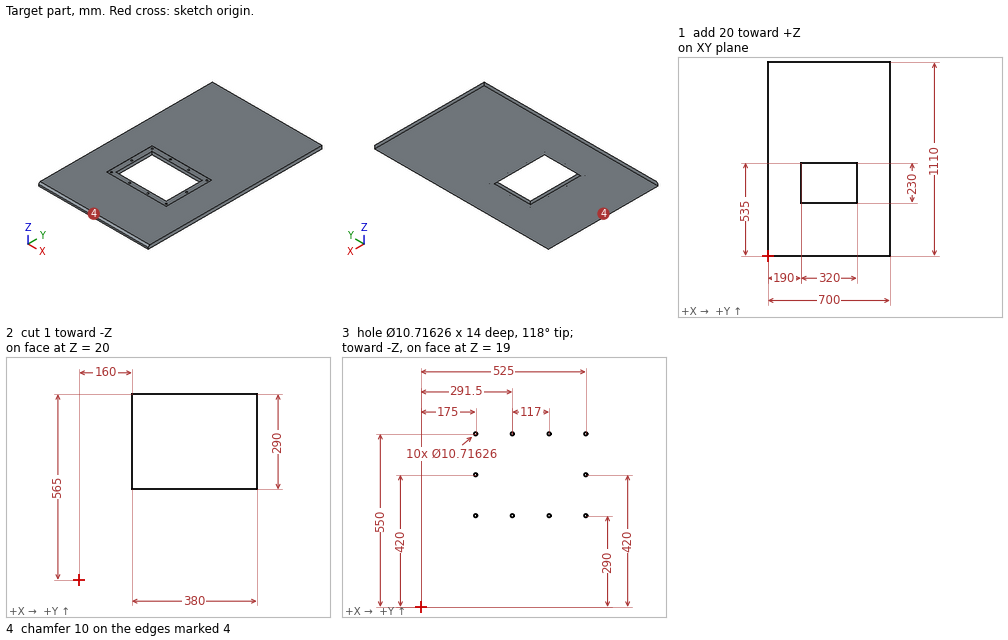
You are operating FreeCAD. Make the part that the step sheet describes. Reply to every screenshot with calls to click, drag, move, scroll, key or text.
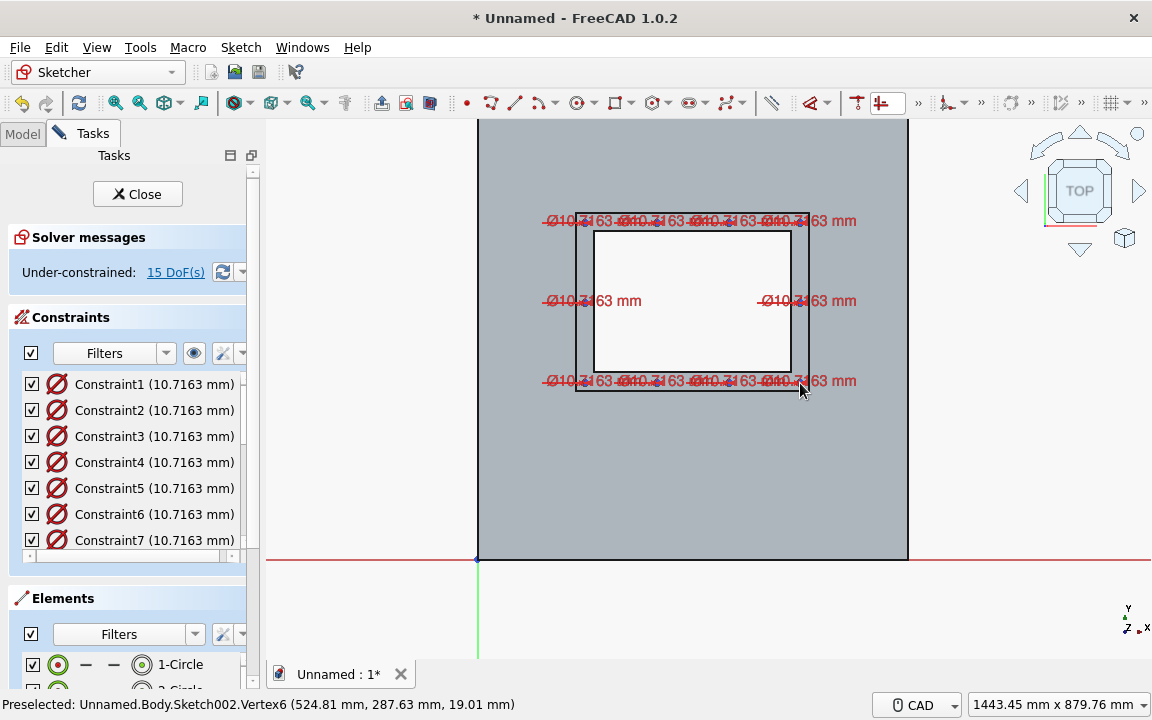
click(729, 223)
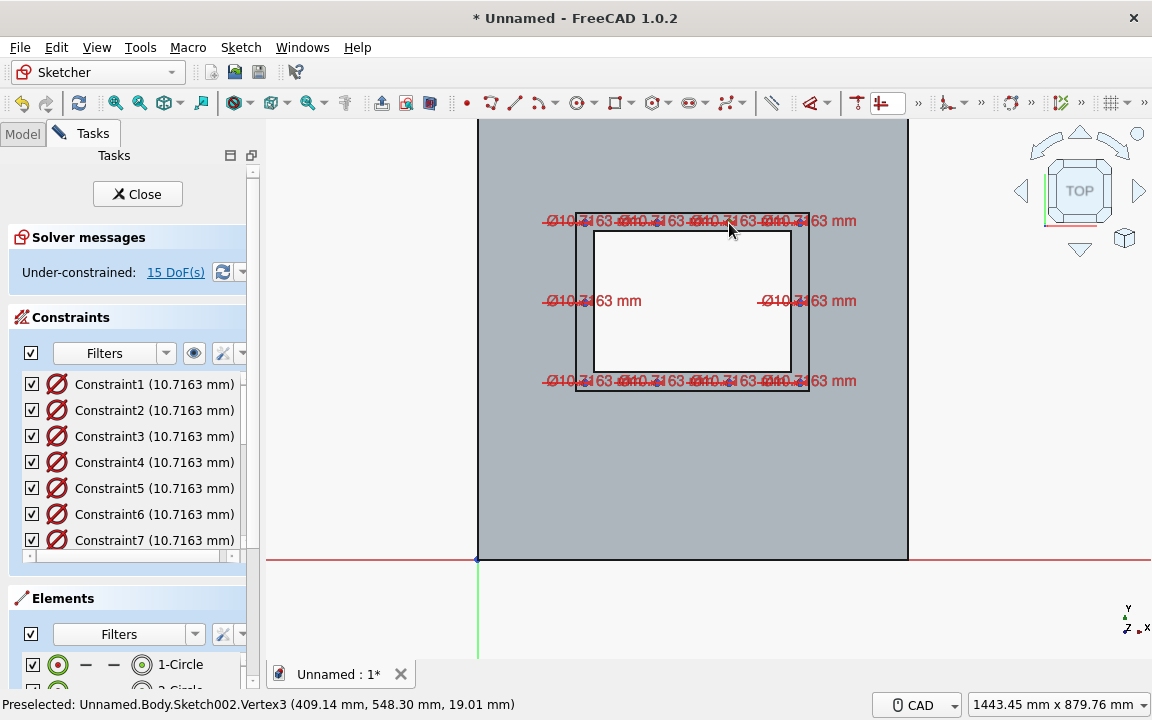
click(729, 383)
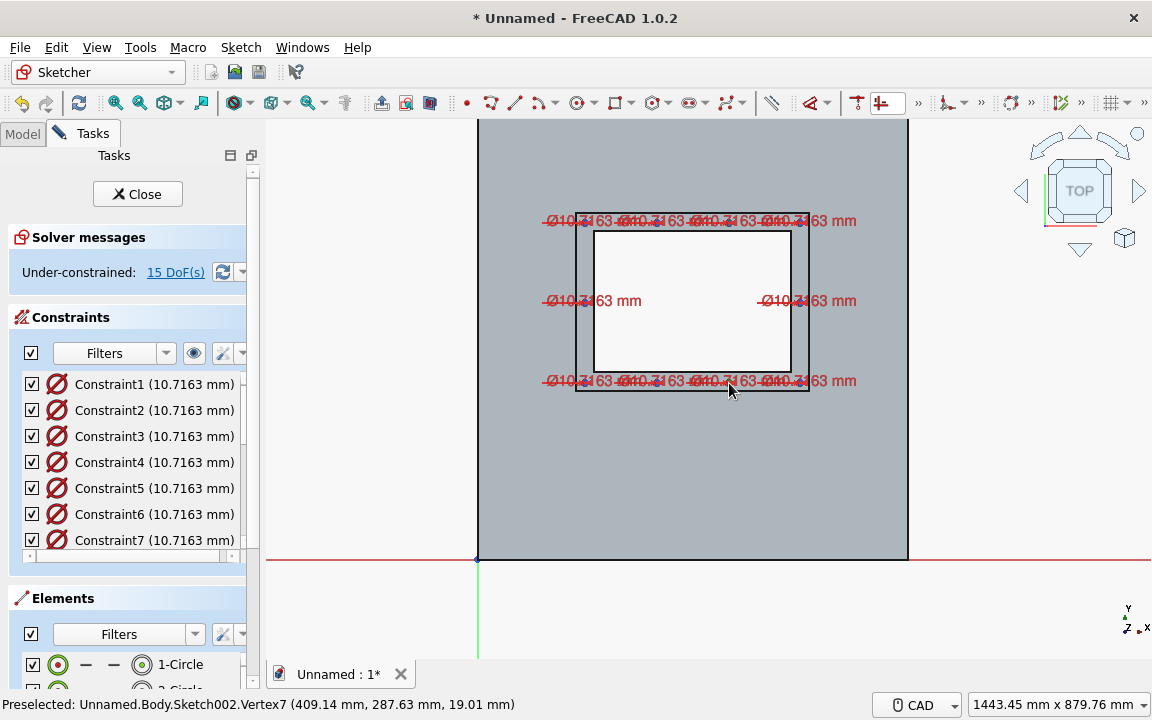
key(v)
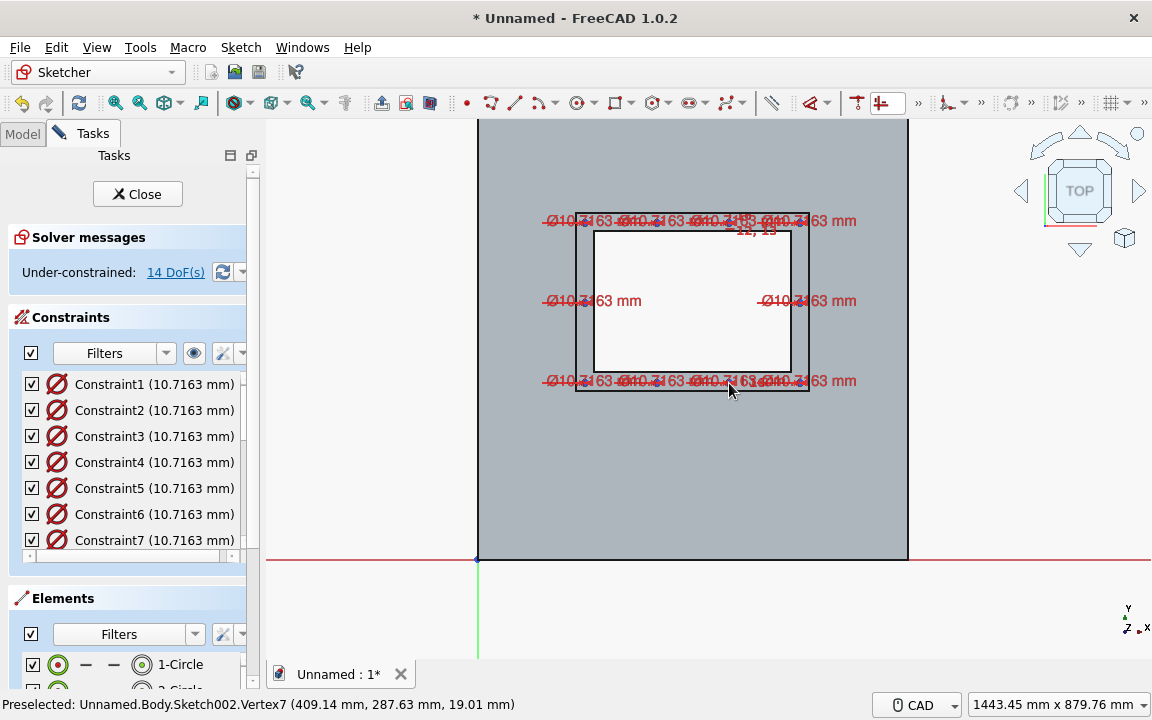
click(800, 383)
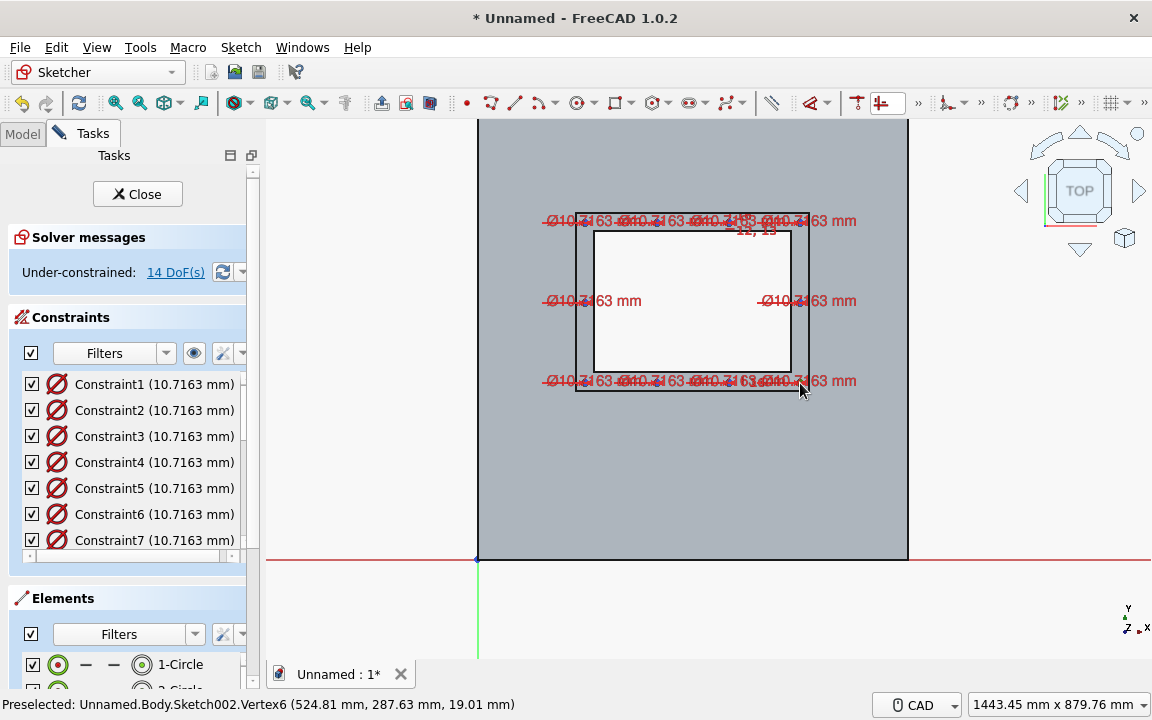
click(729, 383)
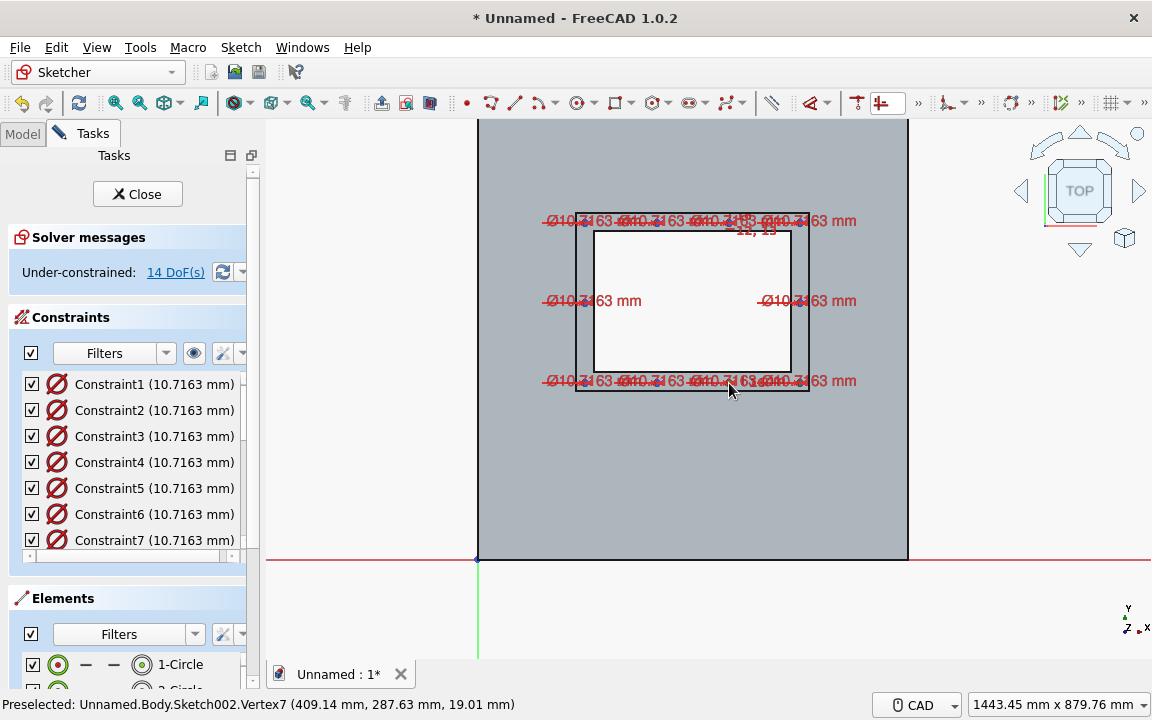
click(900, 104)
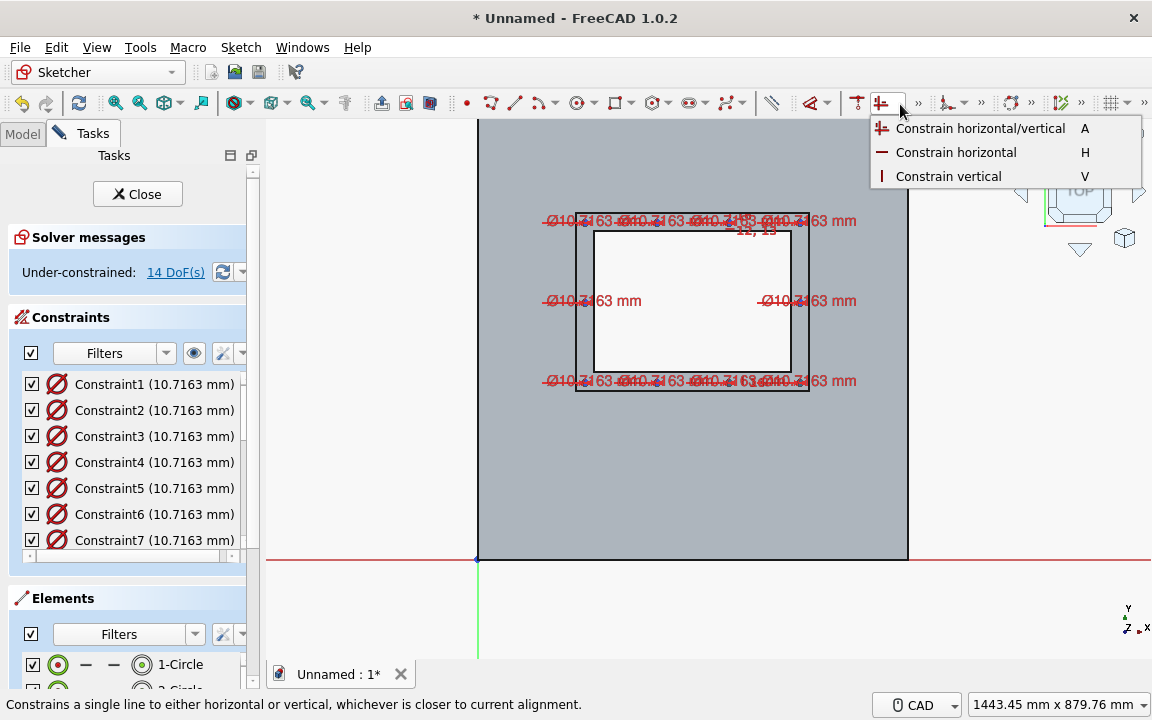
click(1006, 152)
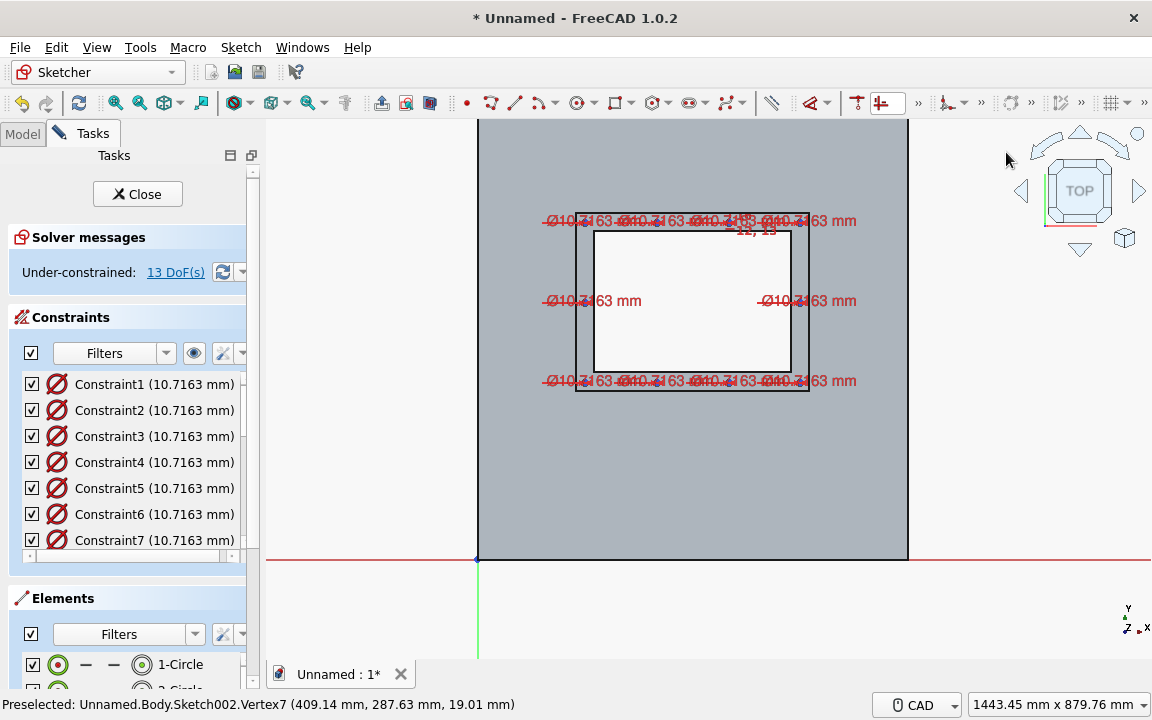
click(657, 223)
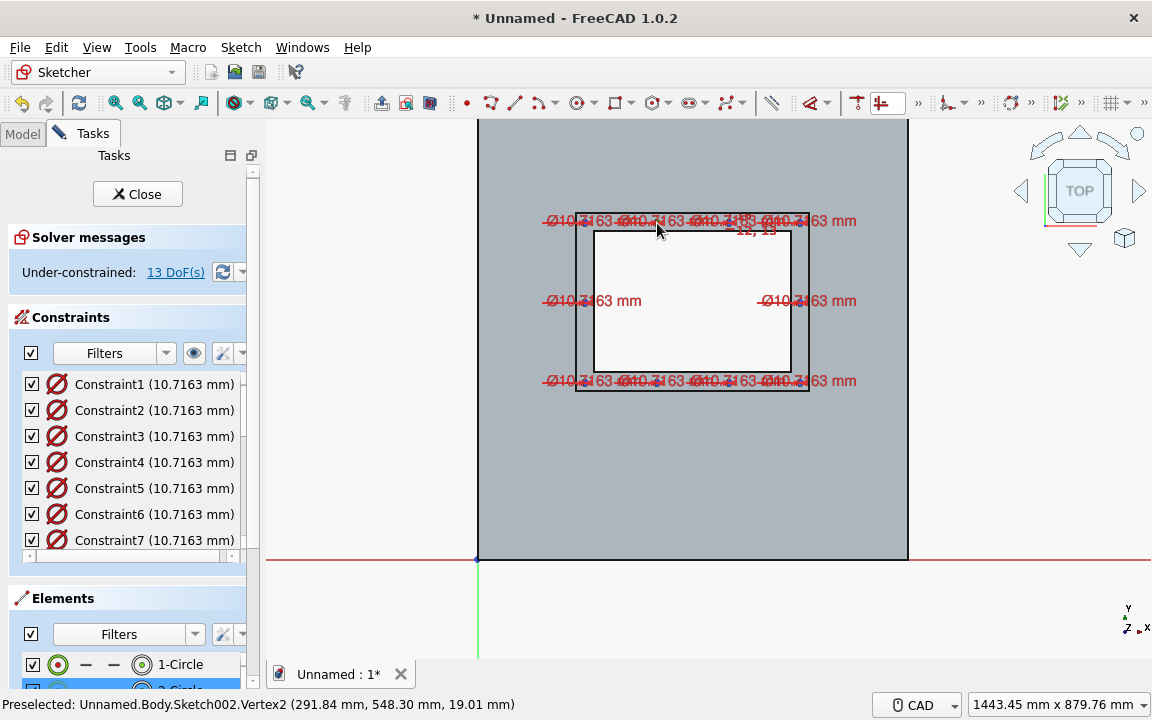
click(657, 383)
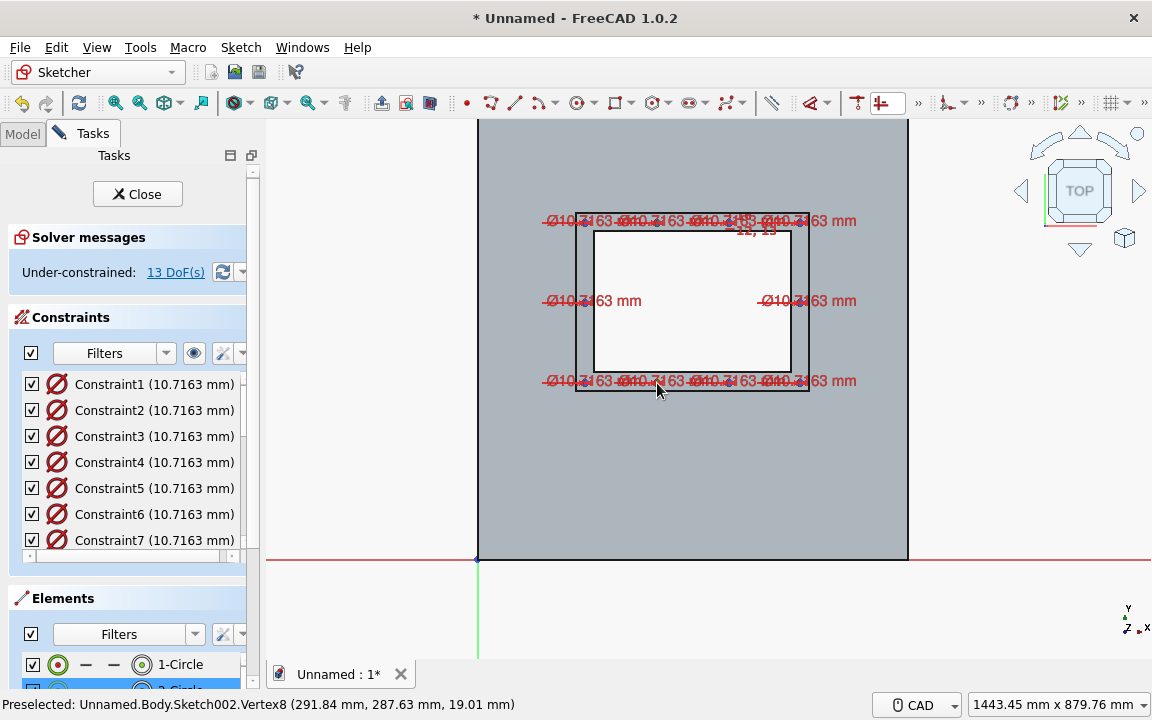
click(900, 104)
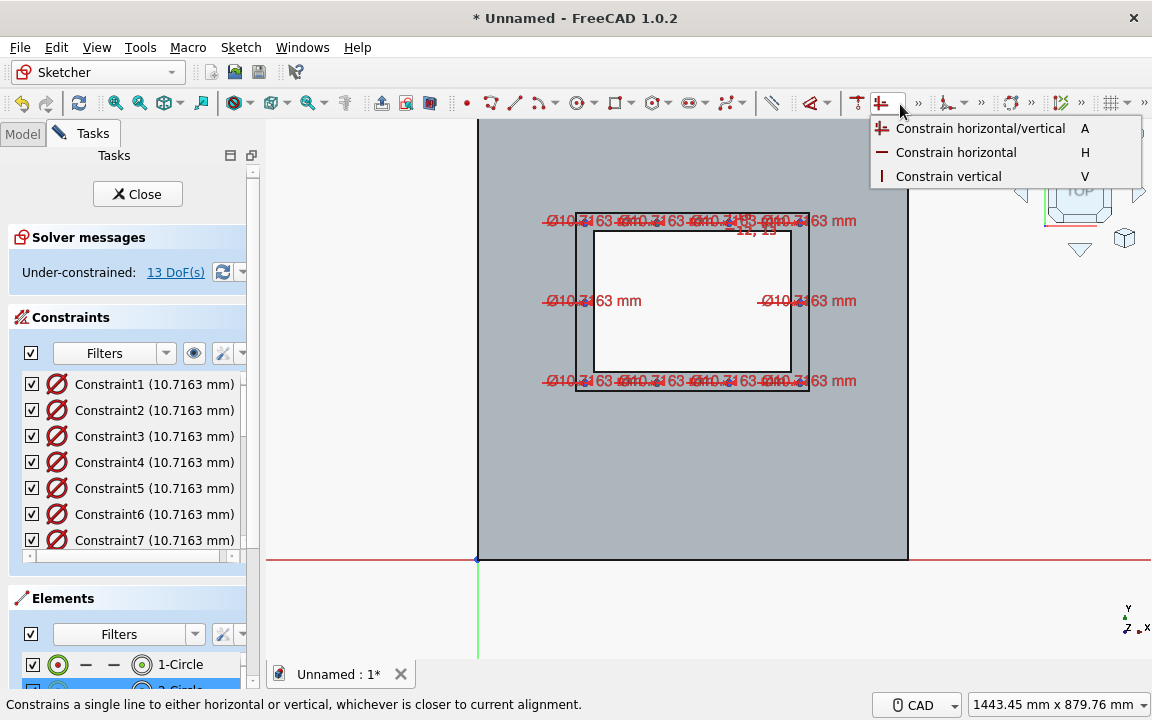
click(1006, 176)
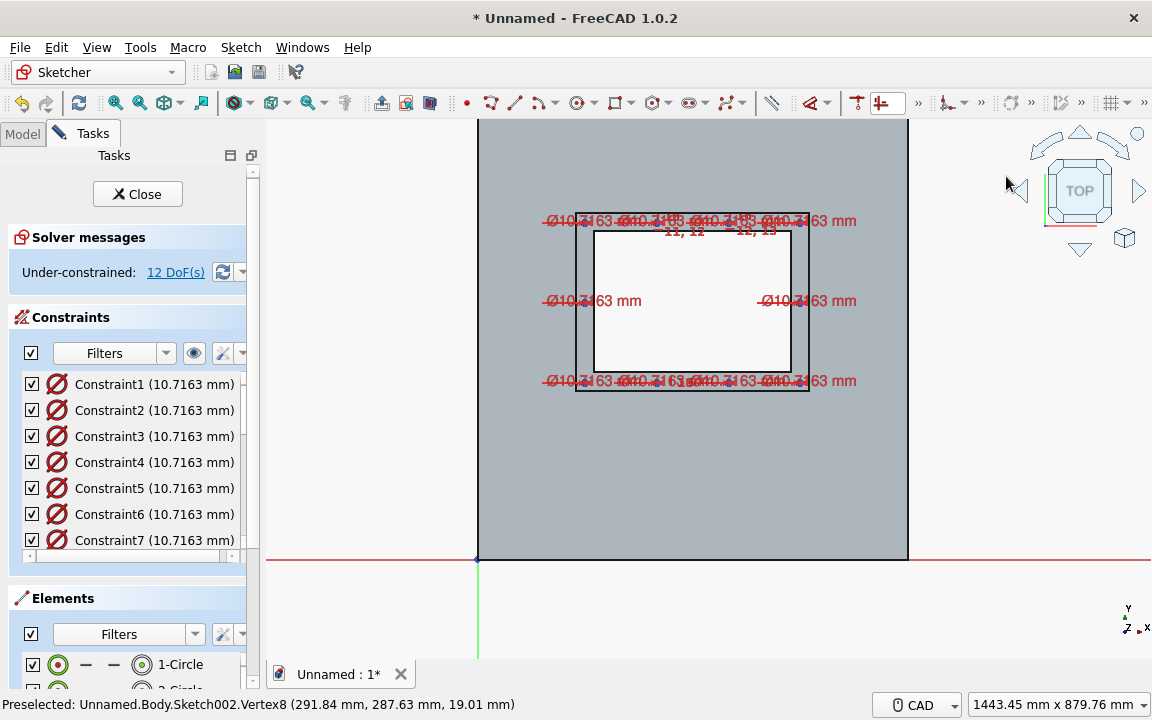
click(729, 383)